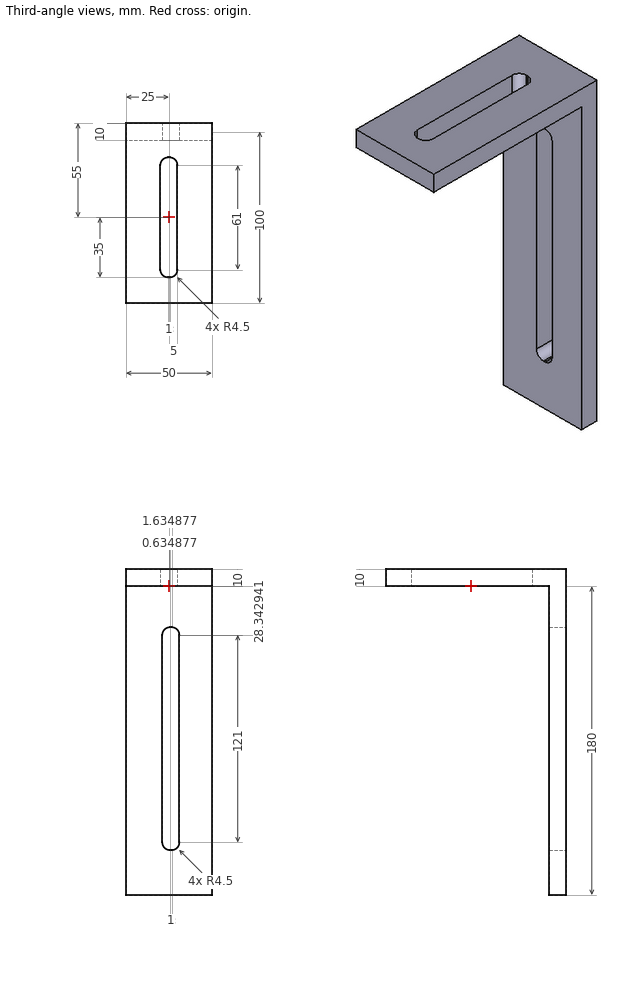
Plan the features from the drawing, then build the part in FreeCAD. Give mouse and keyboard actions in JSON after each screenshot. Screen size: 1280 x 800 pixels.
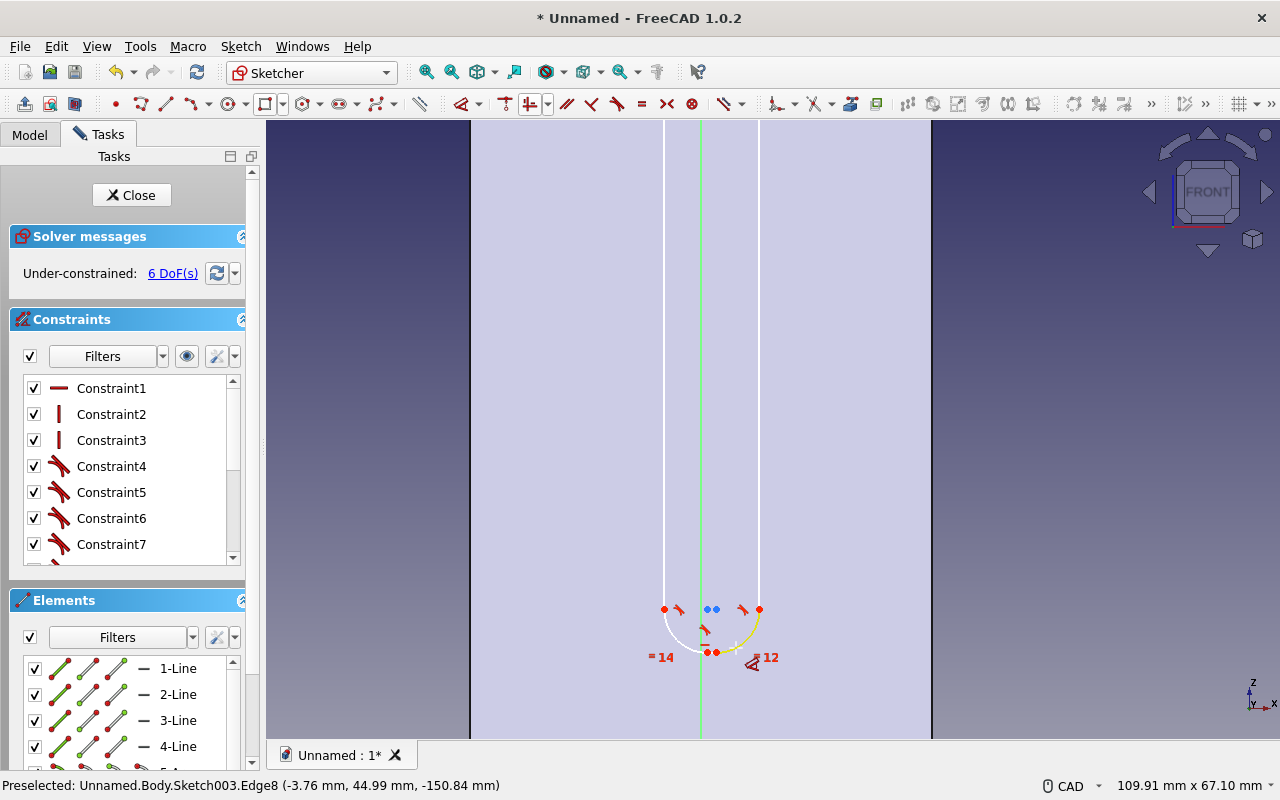
{"action": "left_click", "coordinate": [736, 648]}
{"action": "left_click", "coordinate": [751, 676]}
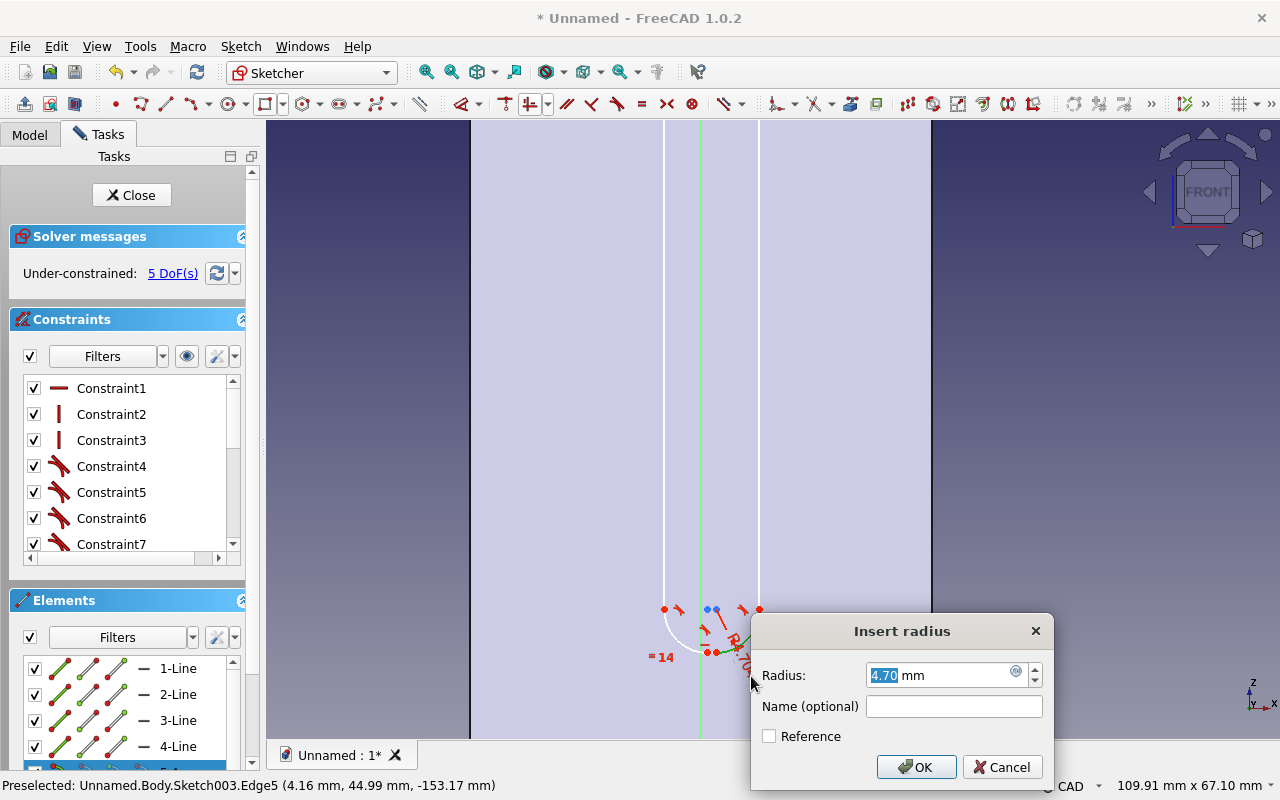
{"action": "type", "text": "4.5"}
{"action": "key", "text": "Return"}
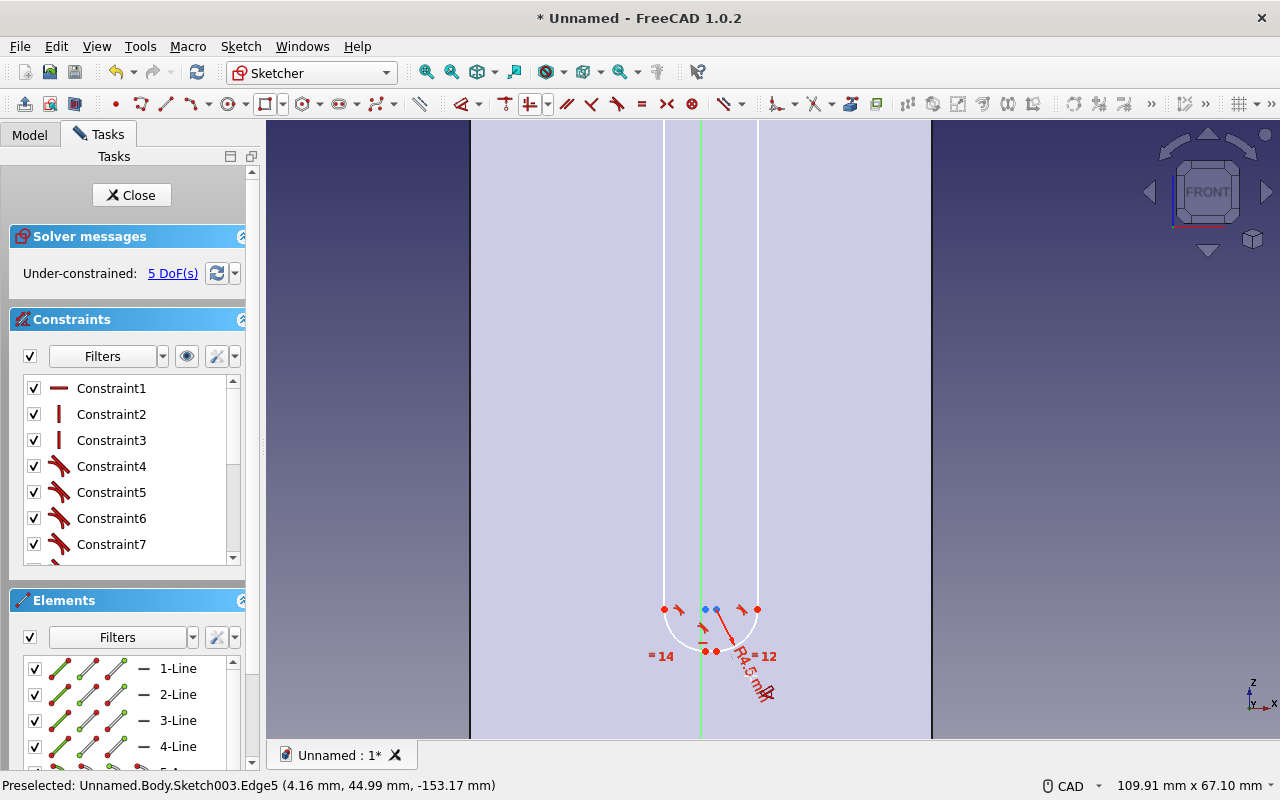
{"action": "scroll", "coordinate": [711, 651], "scroll_direction": "up", "scroll_amount": 8}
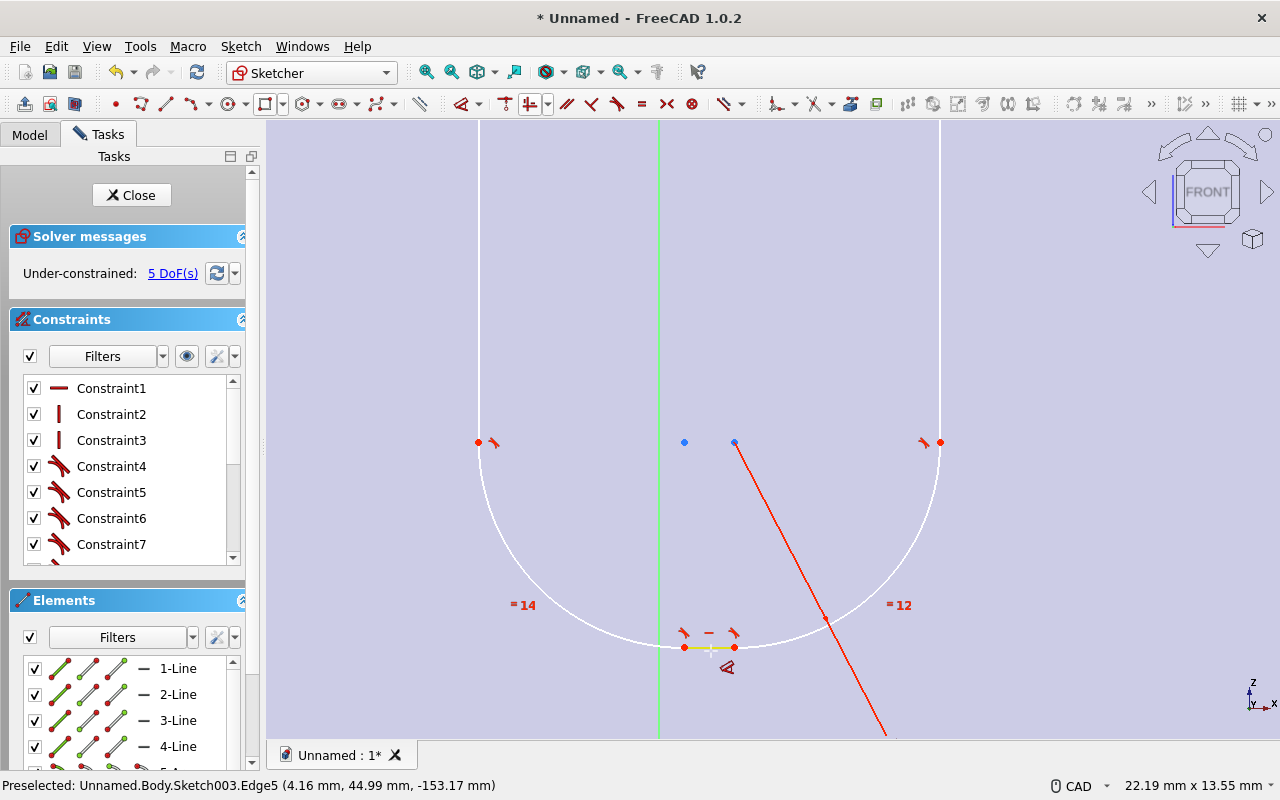
{"action": "left_click", "coordinate": [709, 648]}
{"action": "left_click", "coordinate": [709, 682]}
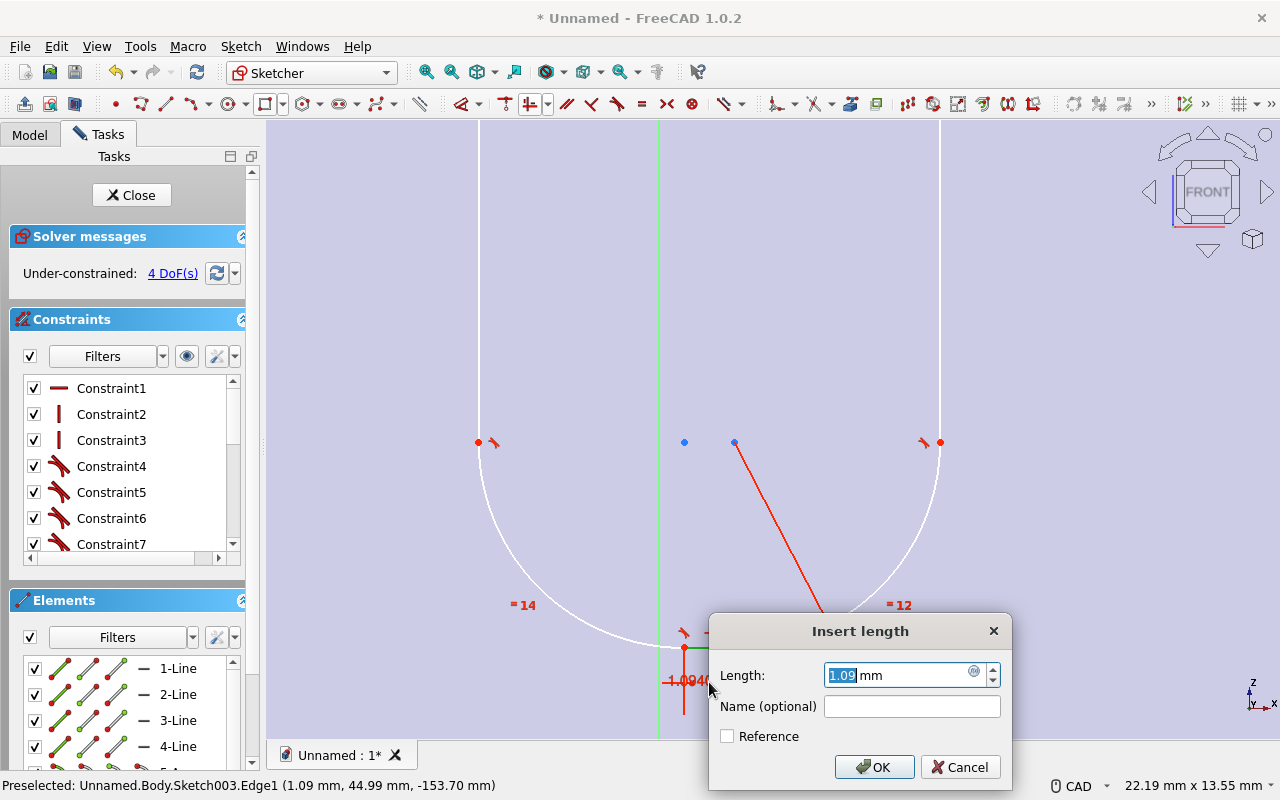
{"action": "type", "text": "1"}
{"action": "key", "text": "Return"}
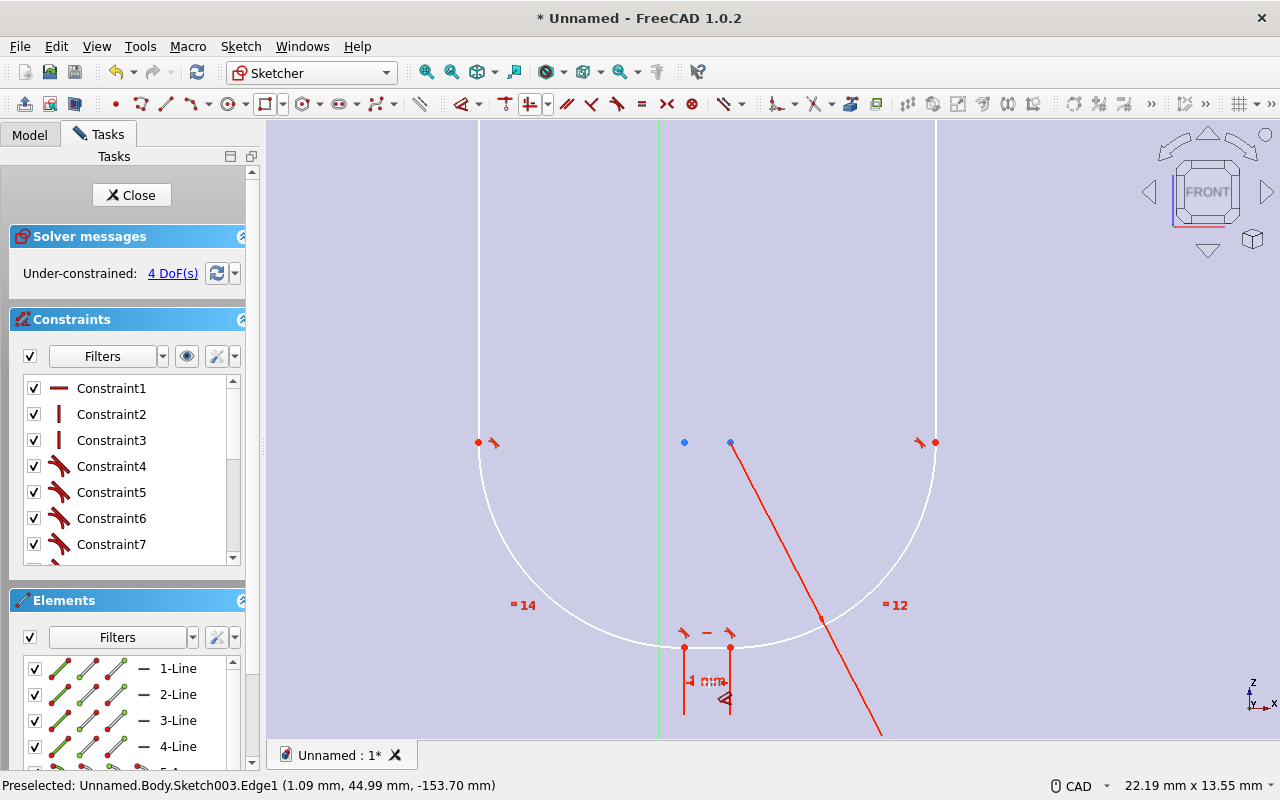
{"action": "scroll", "coordinate": [704, 643], "scroll_direction": "down", "scroll_amount": 14}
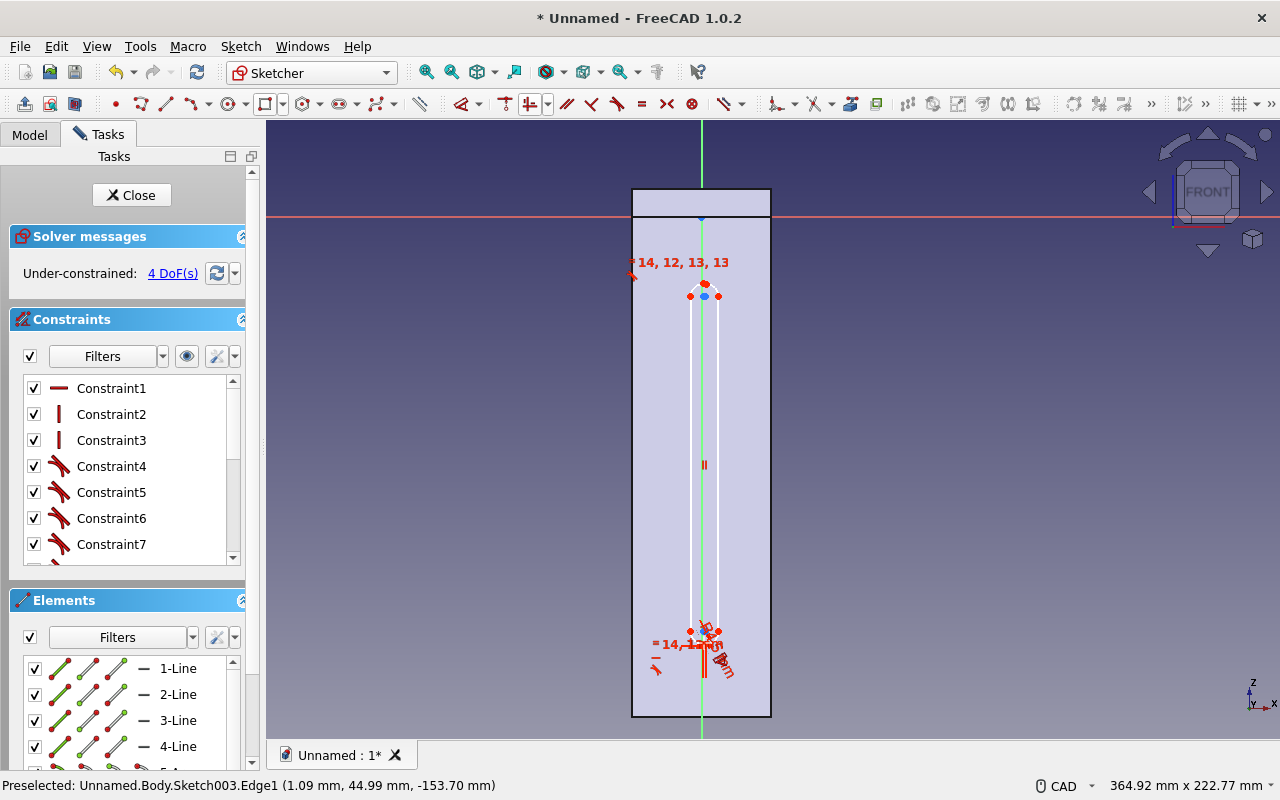
{"action": "left_click", "coordinate": [718, 531]}
{"action": "left_click", "coordinate": [752, 464]}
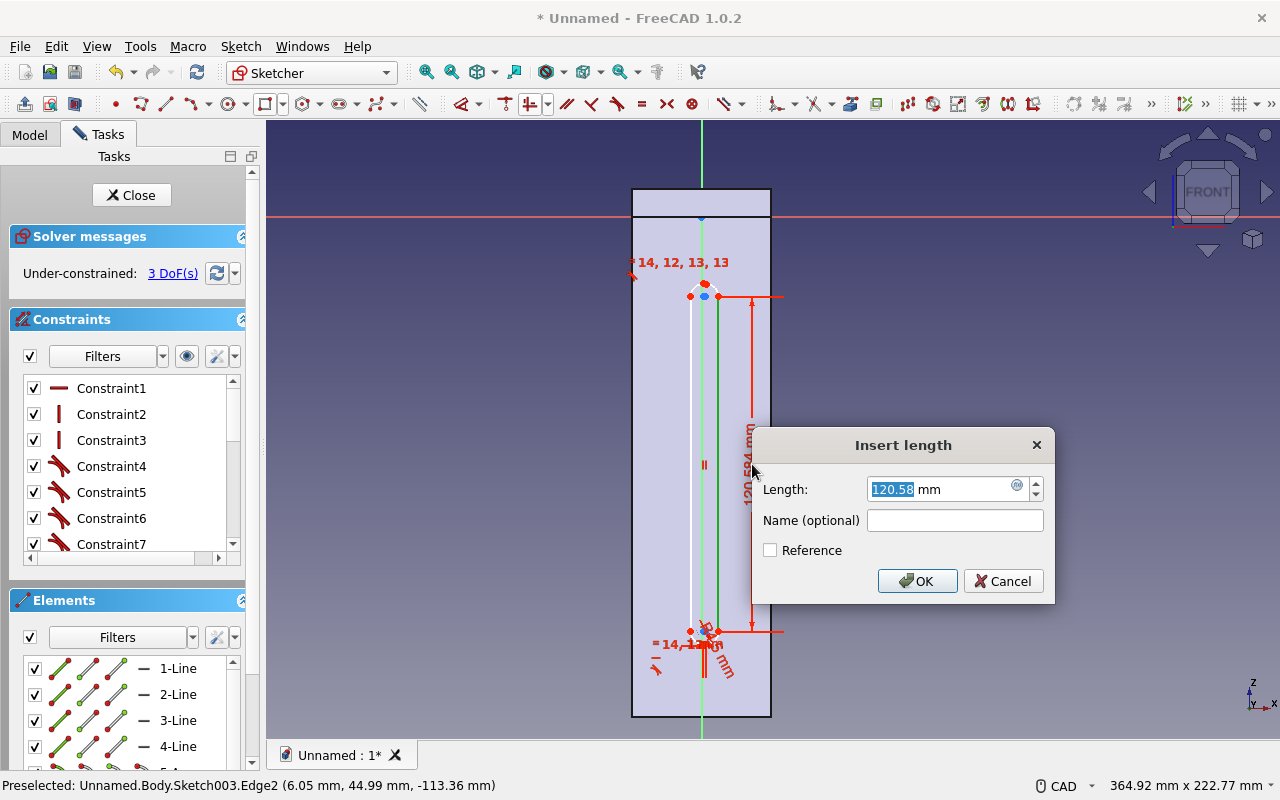
{"action": "type", "text": "121"}
{"action": "key", "text": "Return"}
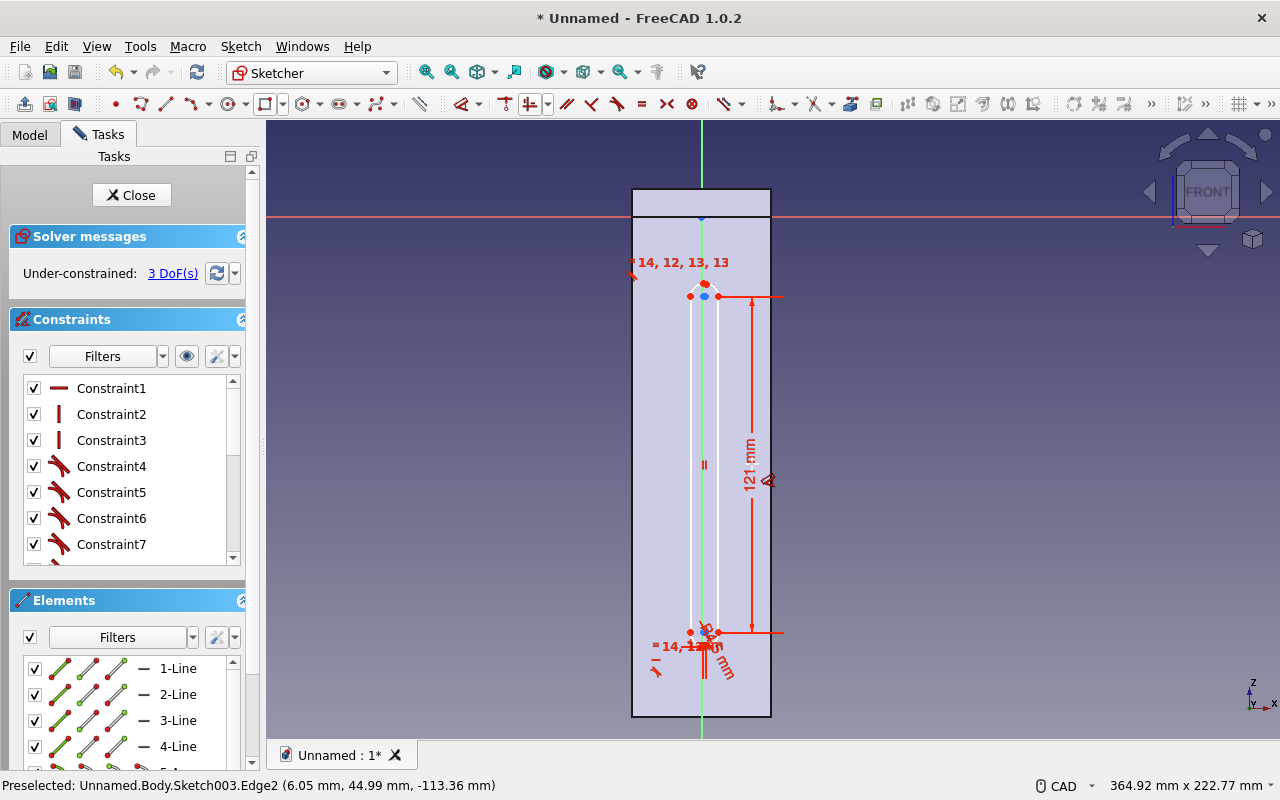
{"action": "scroll", "coordinate": [703, 645], "scroll_direction": "up", "scroll_amount": 16}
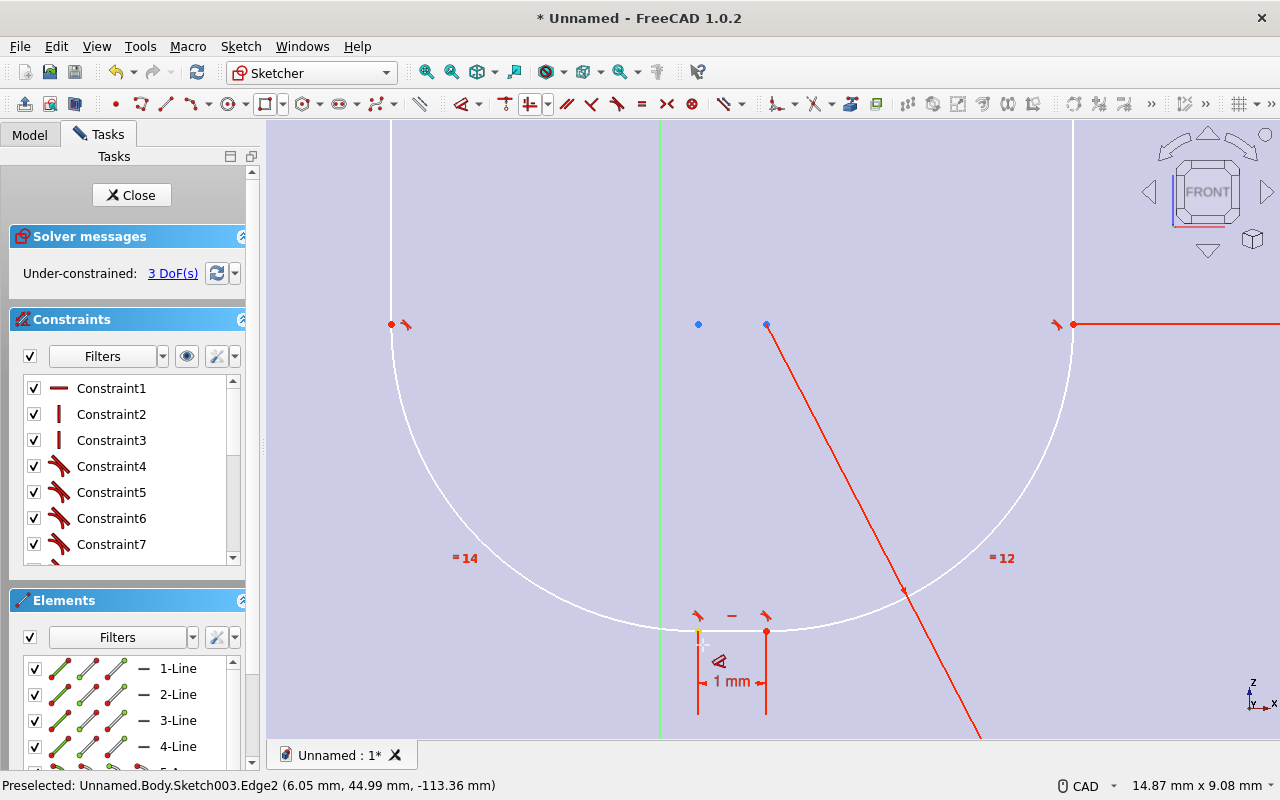
{"action": "left_click", "coordinate": [698, 631]}
{"action": "left_click", "coordinate": [679, 689]}